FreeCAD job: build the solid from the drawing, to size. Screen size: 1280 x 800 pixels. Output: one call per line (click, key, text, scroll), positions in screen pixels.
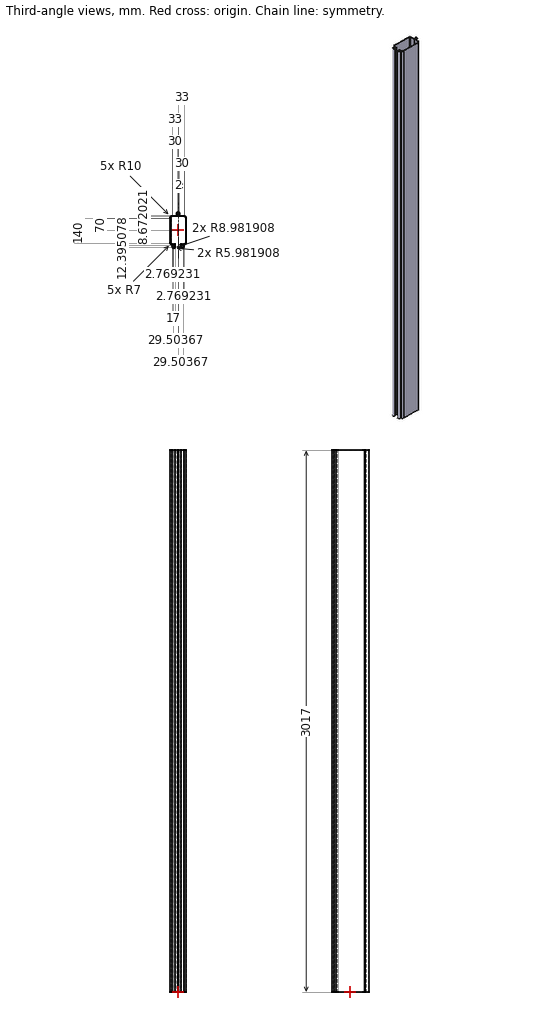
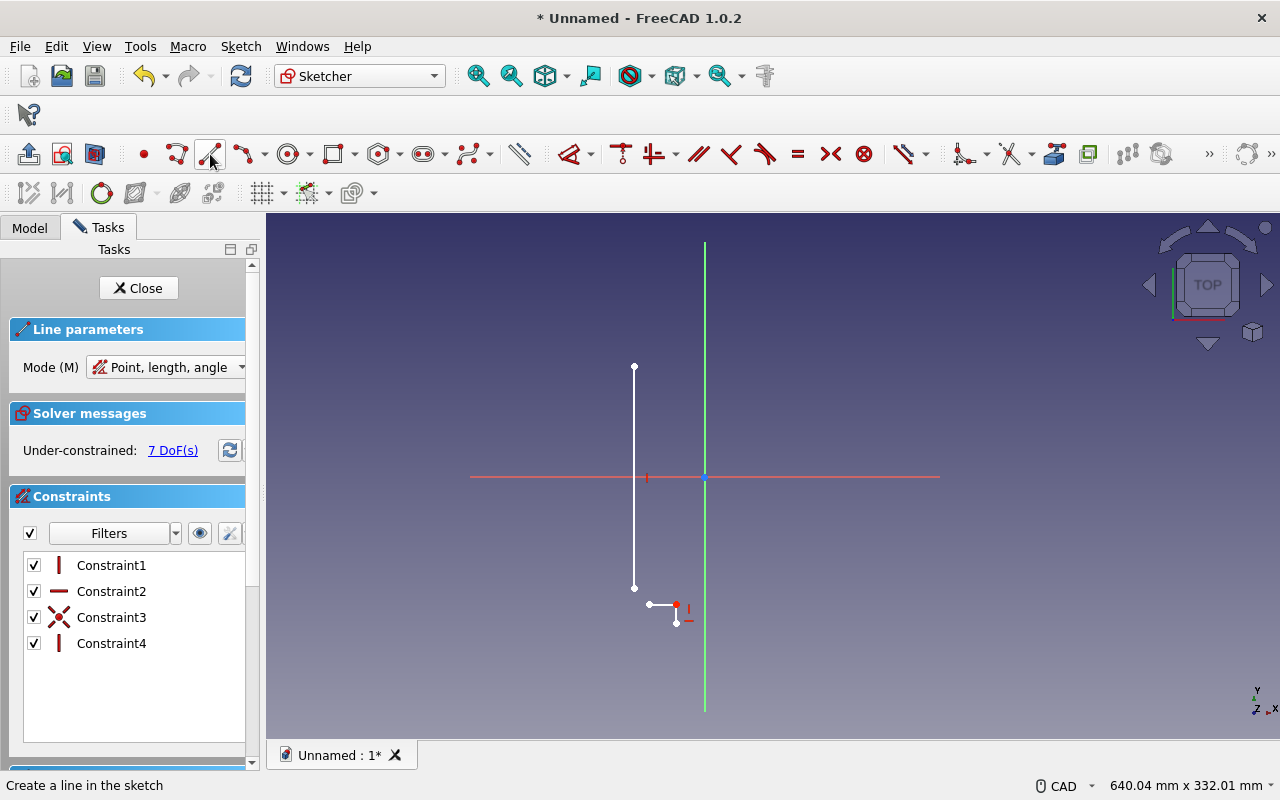
click(658, 620)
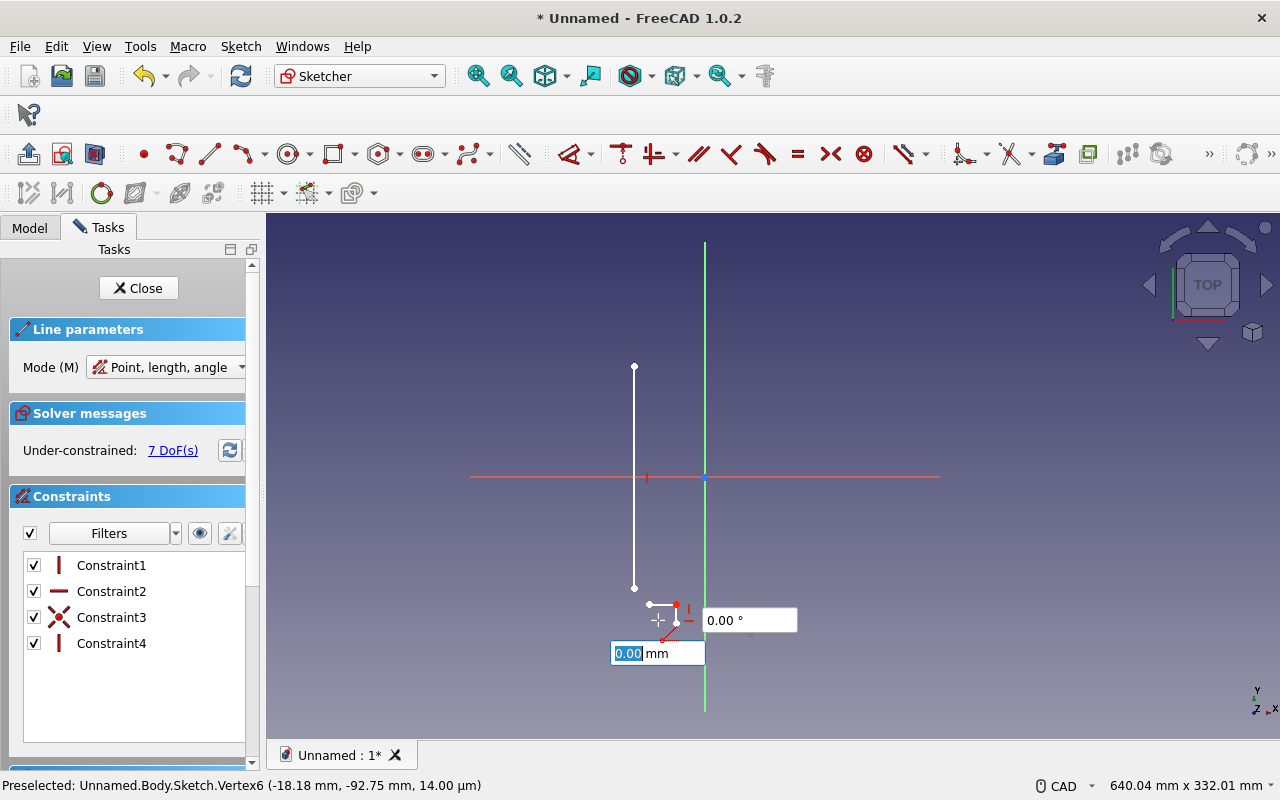
scroll(654, 618, up, 7)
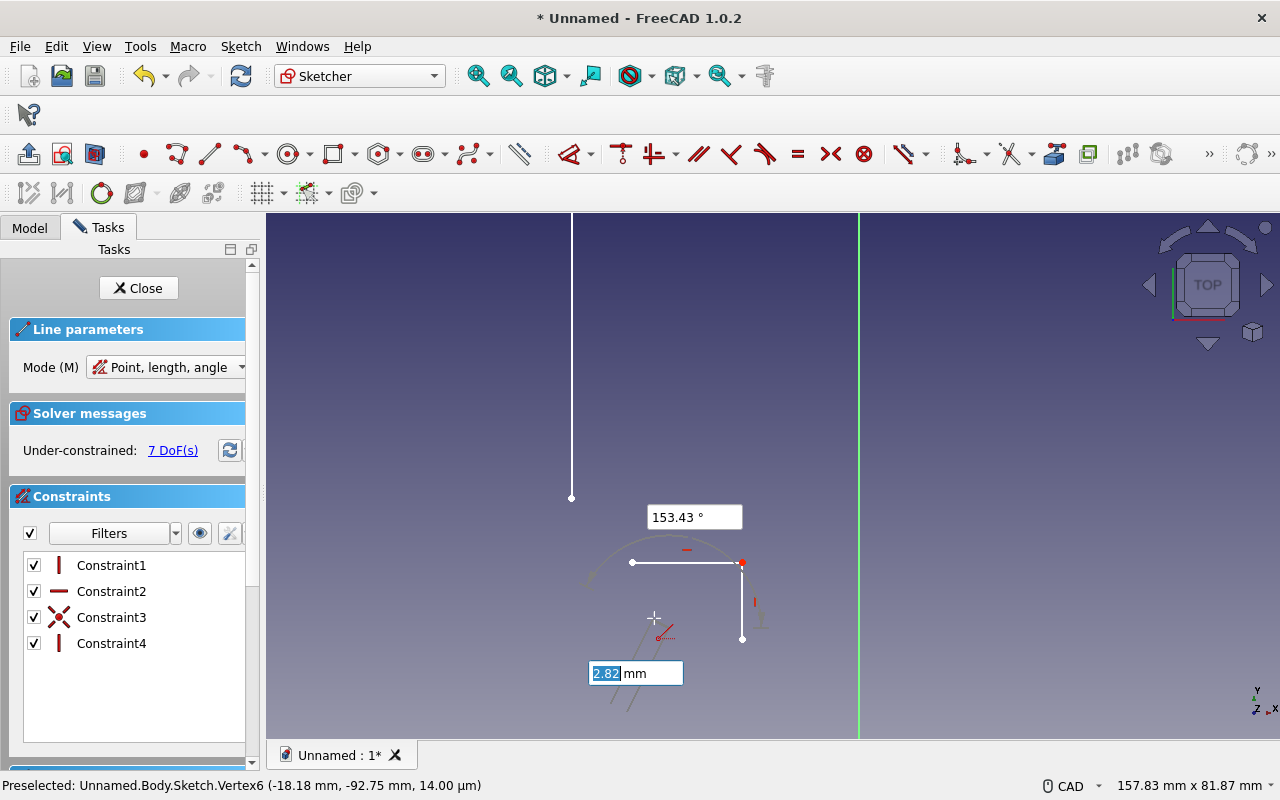
click(651, 615)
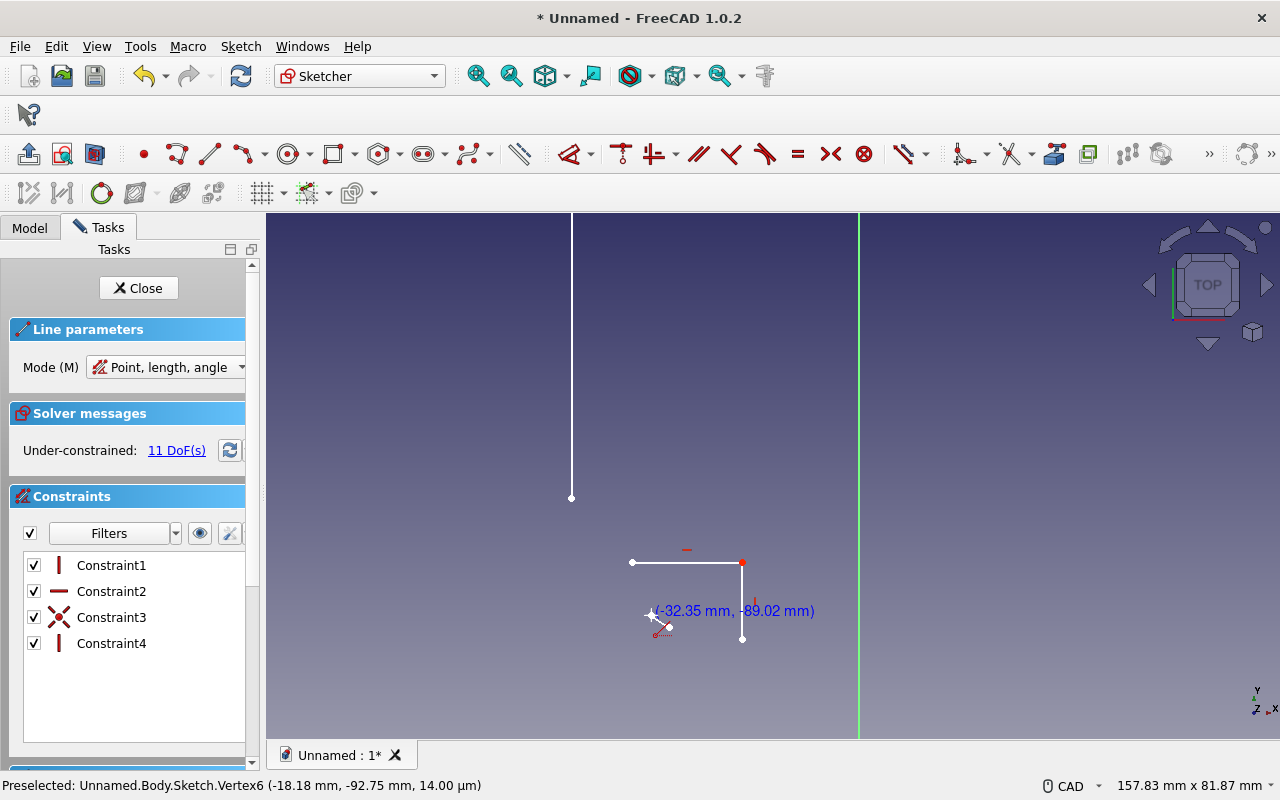
click(177, 154)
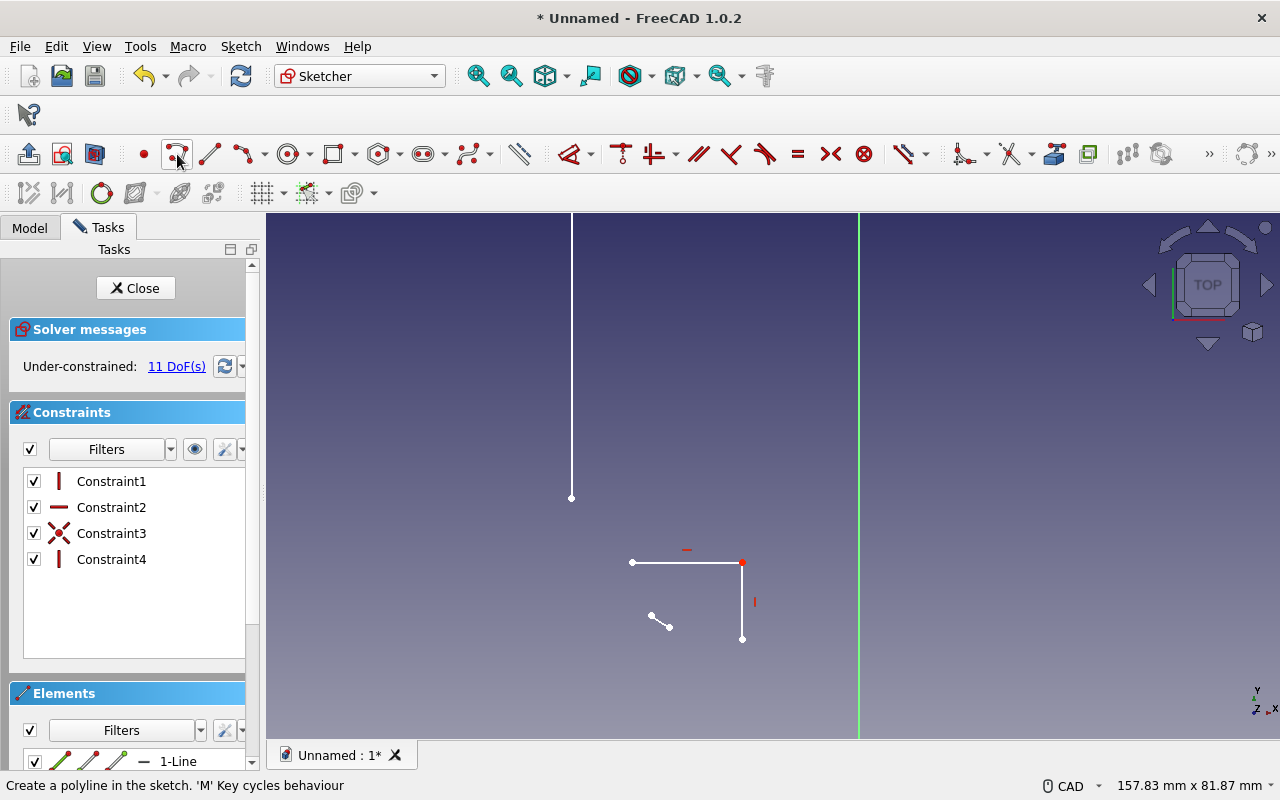
click(762, 638)
click(762, 539)
click(634, 539)
right_click(634, 539)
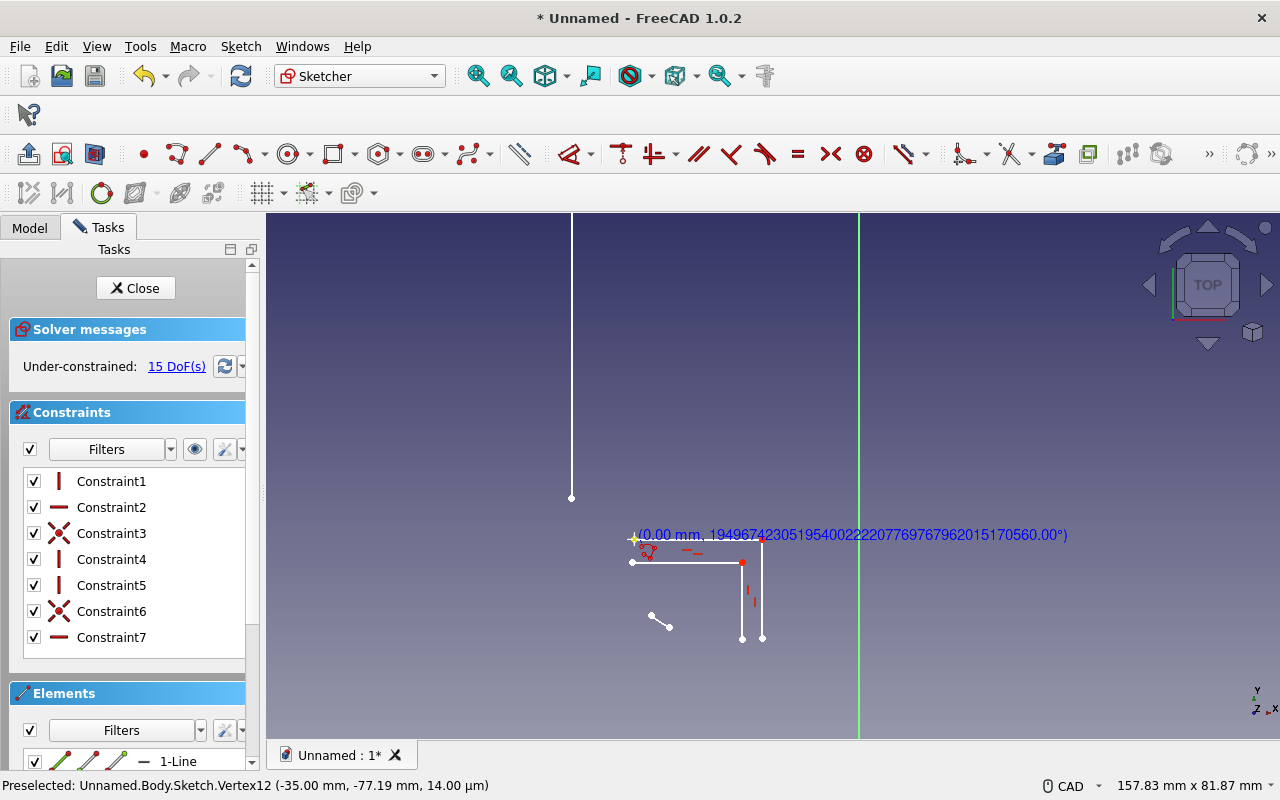
click(210, 154)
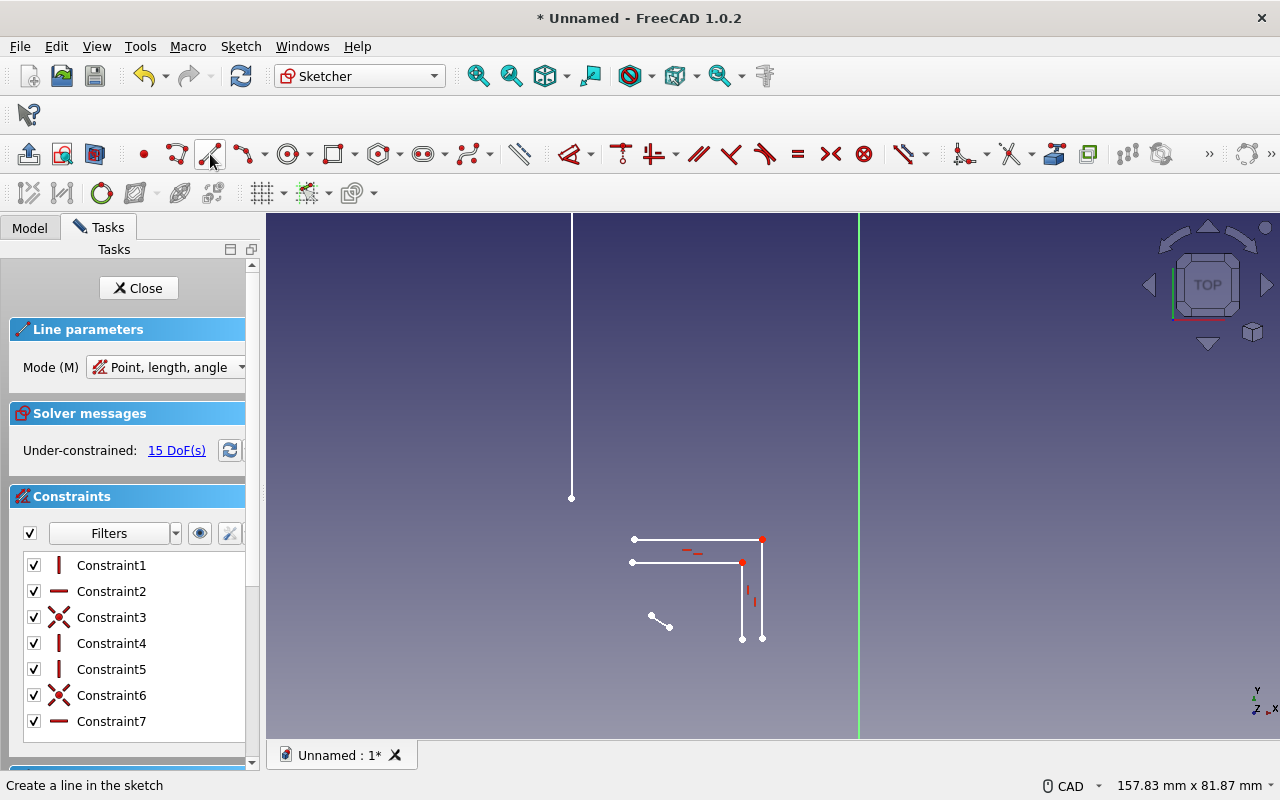
click(589, 494)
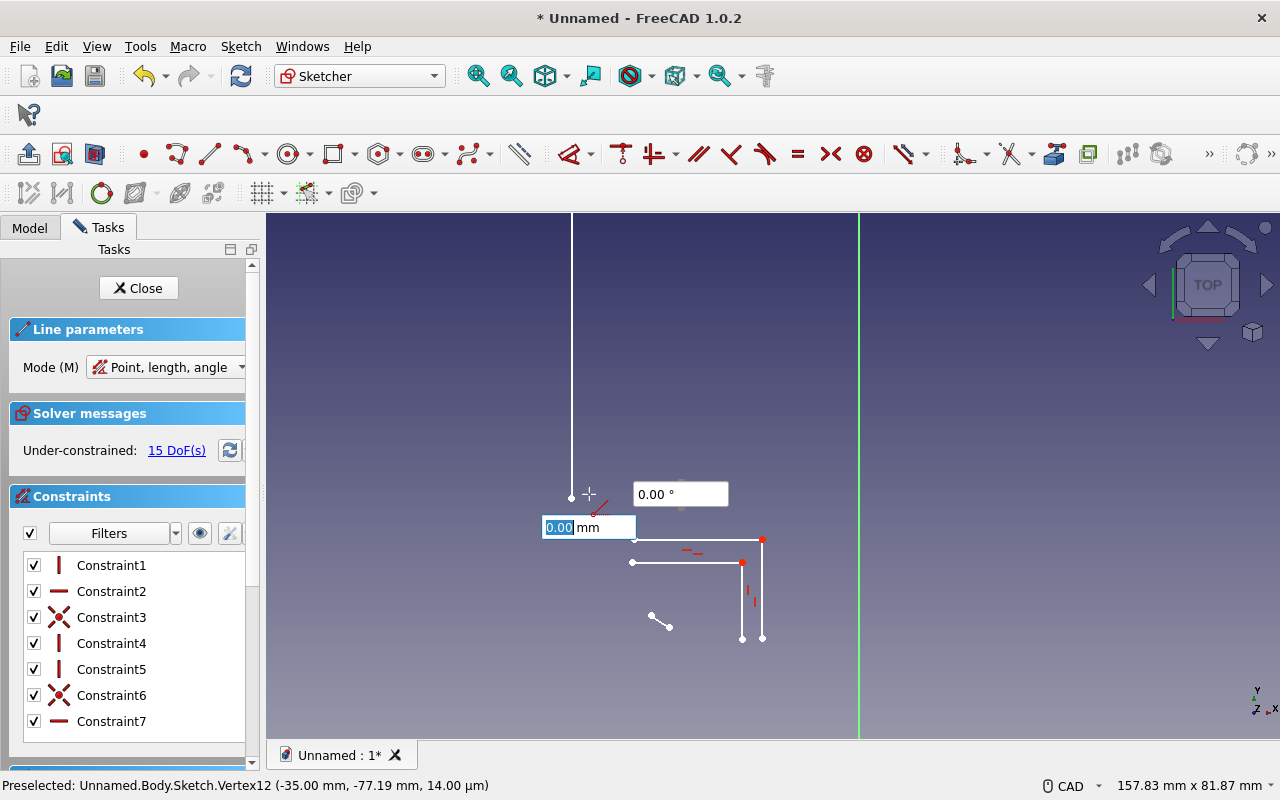
scroll(654, 619, down, 7)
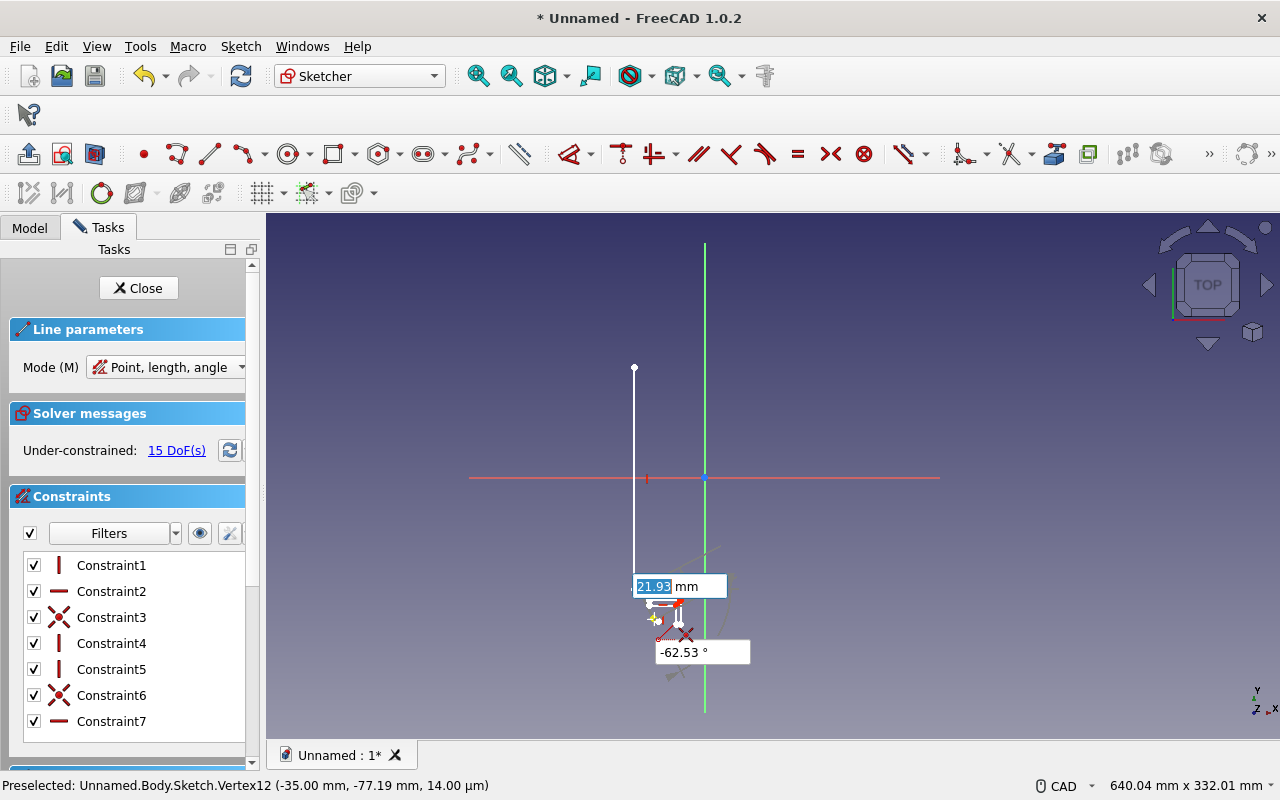
scroll(638, 367, up, 7)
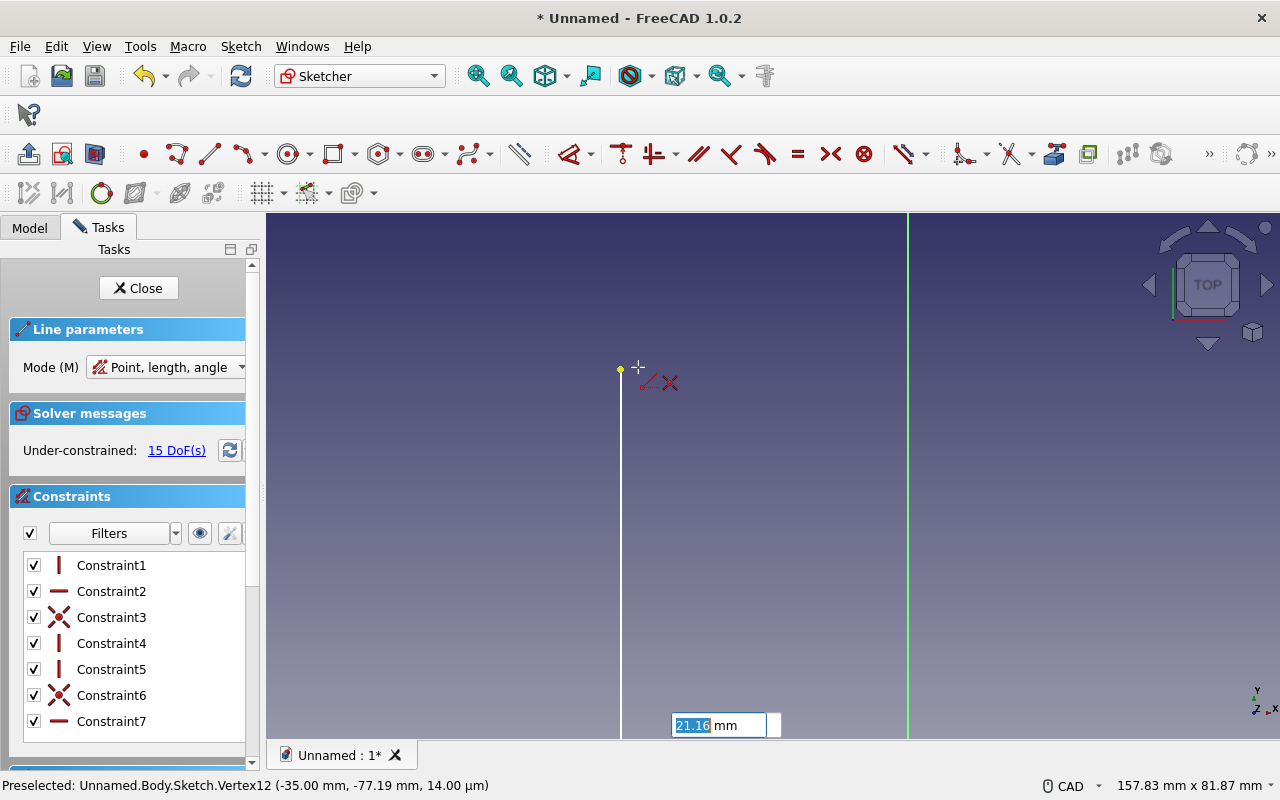
click(638, 366)